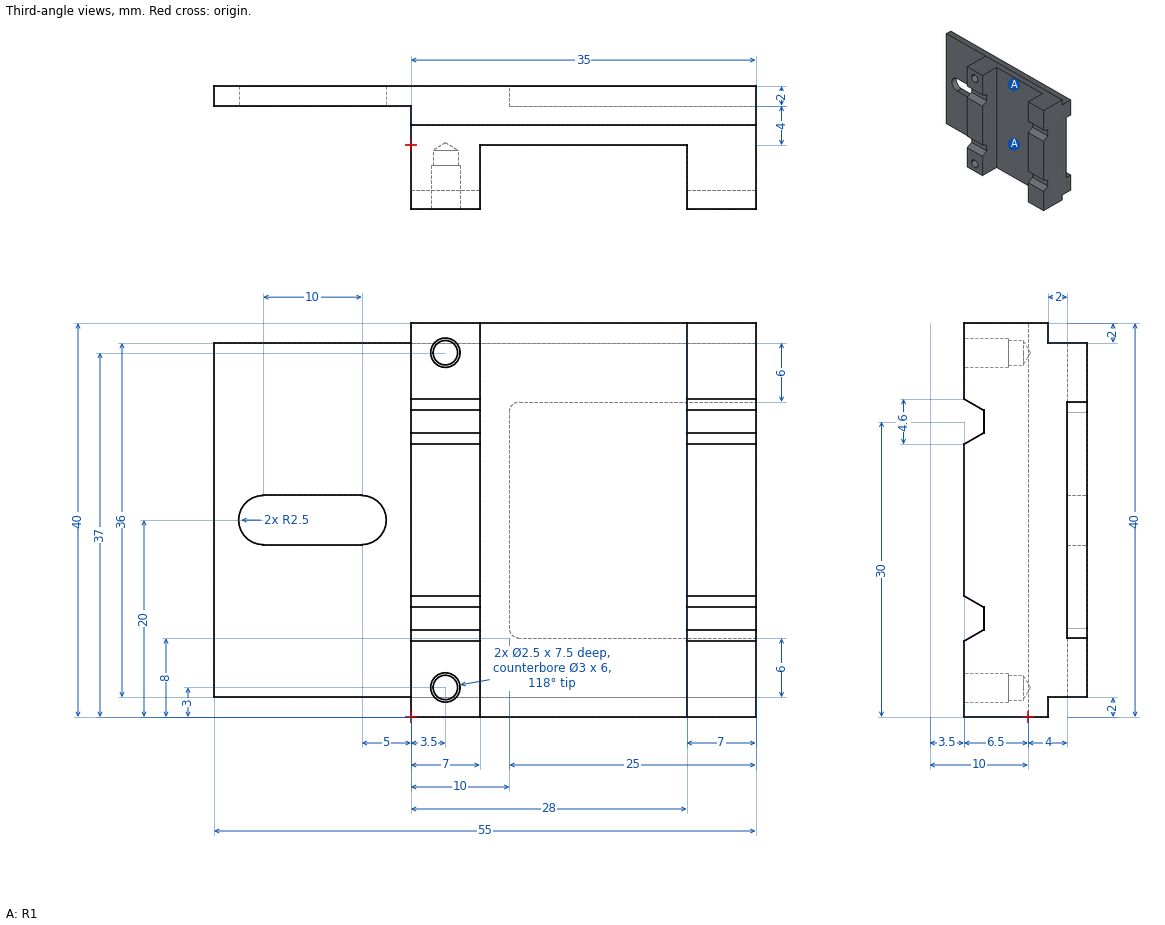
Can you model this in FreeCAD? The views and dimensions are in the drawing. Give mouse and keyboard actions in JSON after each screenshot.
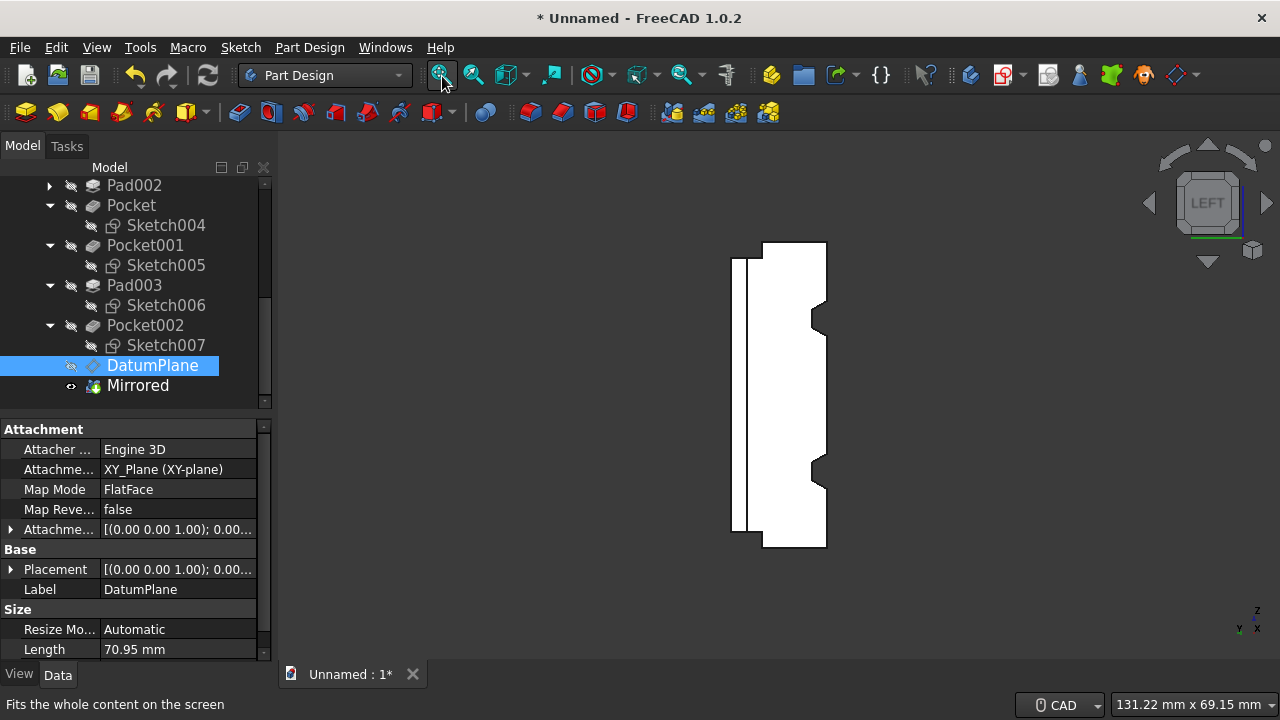
{"action": "key", "text": "0"}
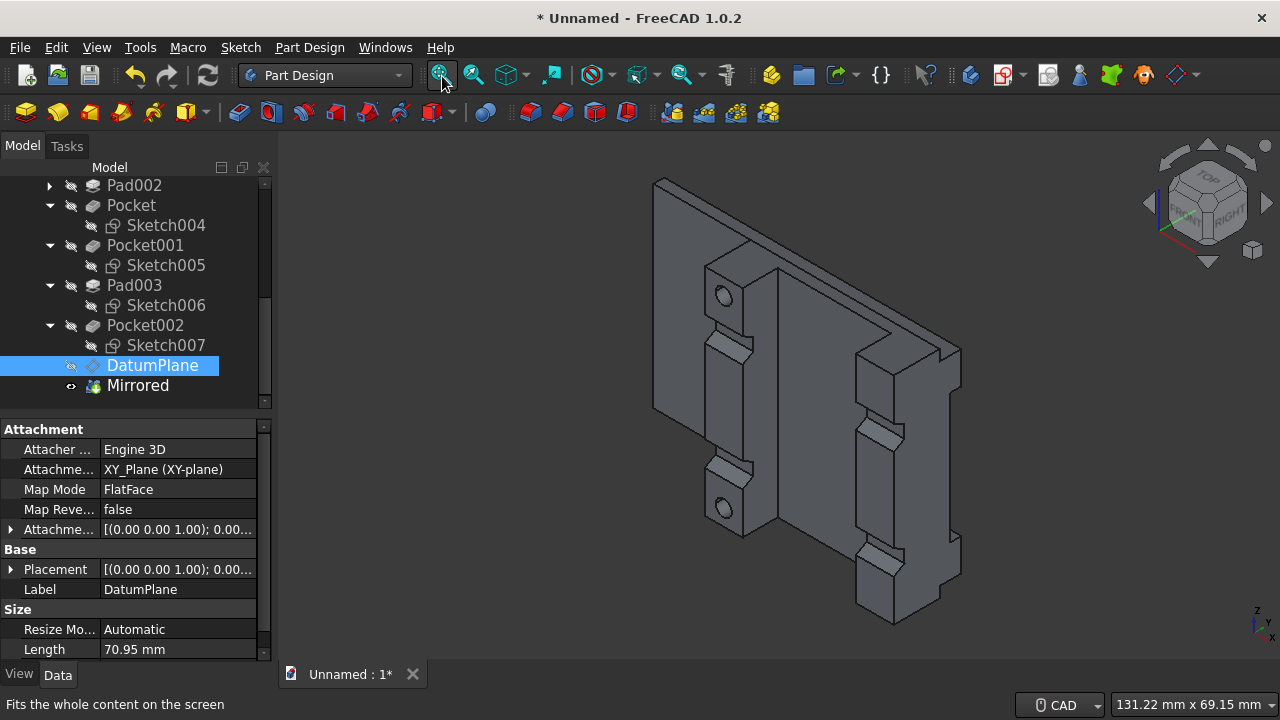
{"action": "scroll", "coordinate": [821, 311], "scroll_direction": "up", "scroll_amount": 5}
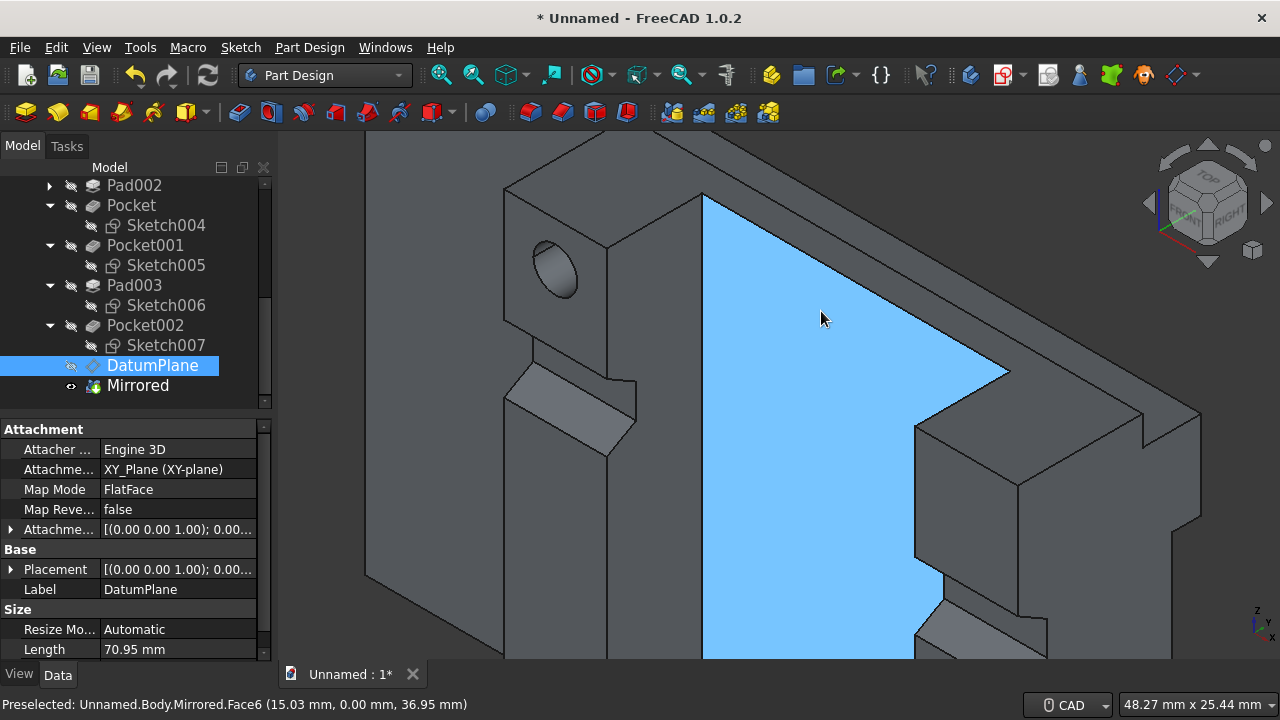
{"action": "left_click", "coordinate": [442, 76]}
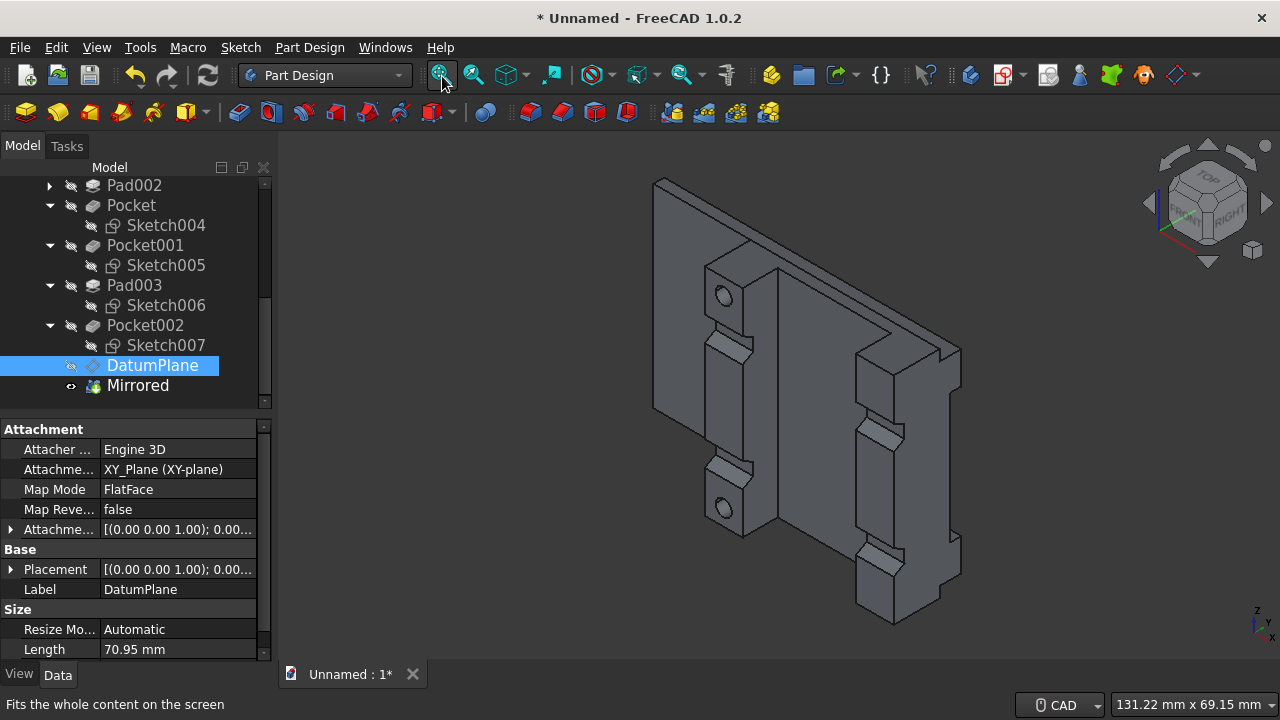
{"action": "key", "text": "2"}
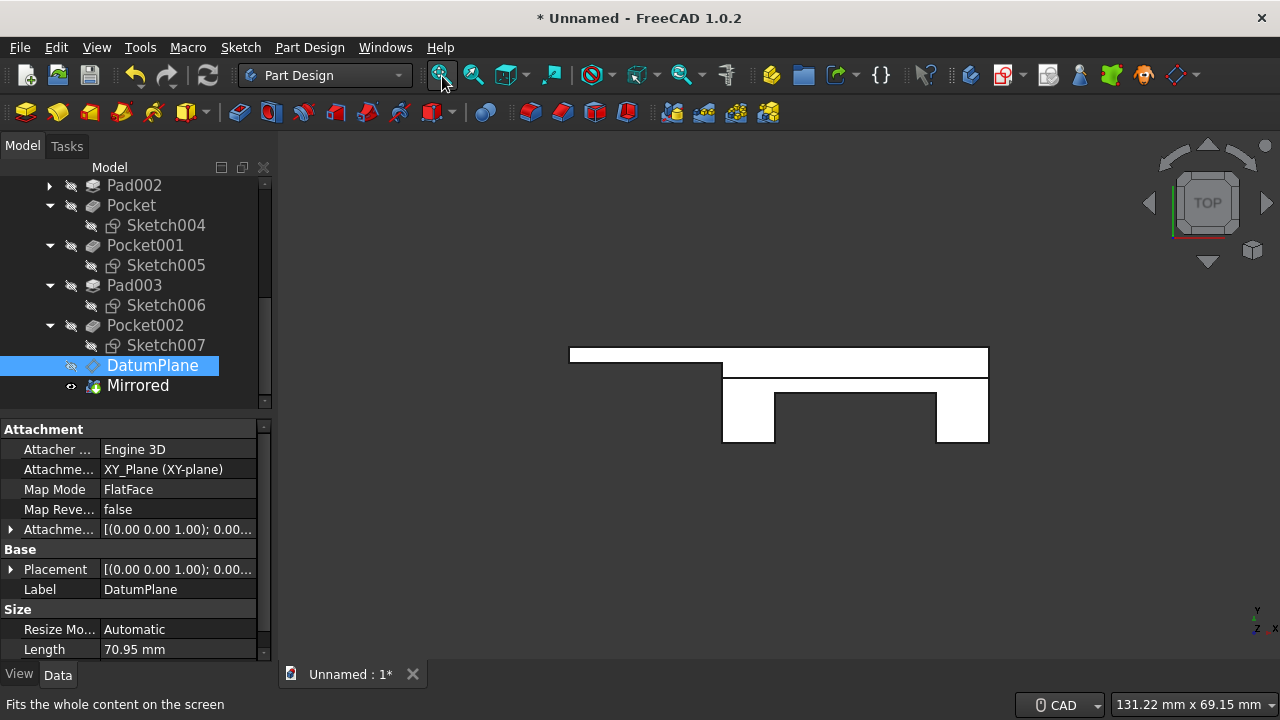
{"action": "left_click", "coordinate": [442, 76]}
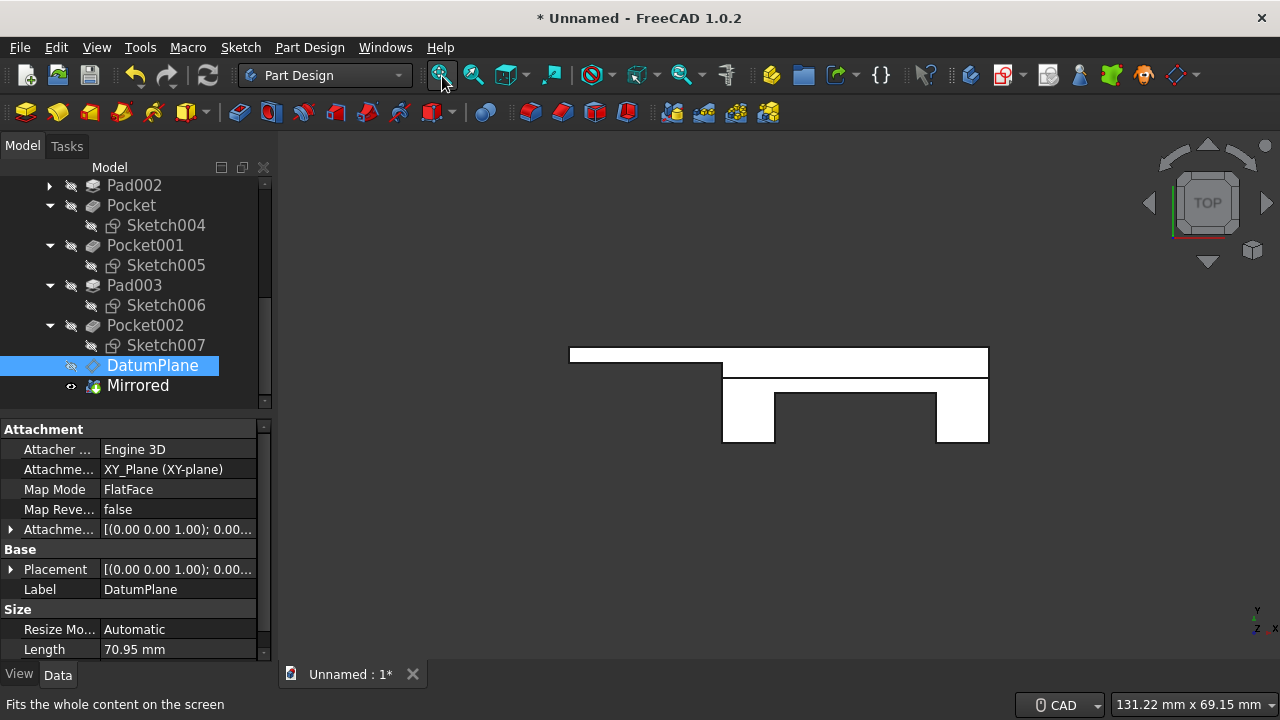
{"action": "scroll", "coordinate": [798, 354], "scroll_direction": "up", "scroll_amount": 5}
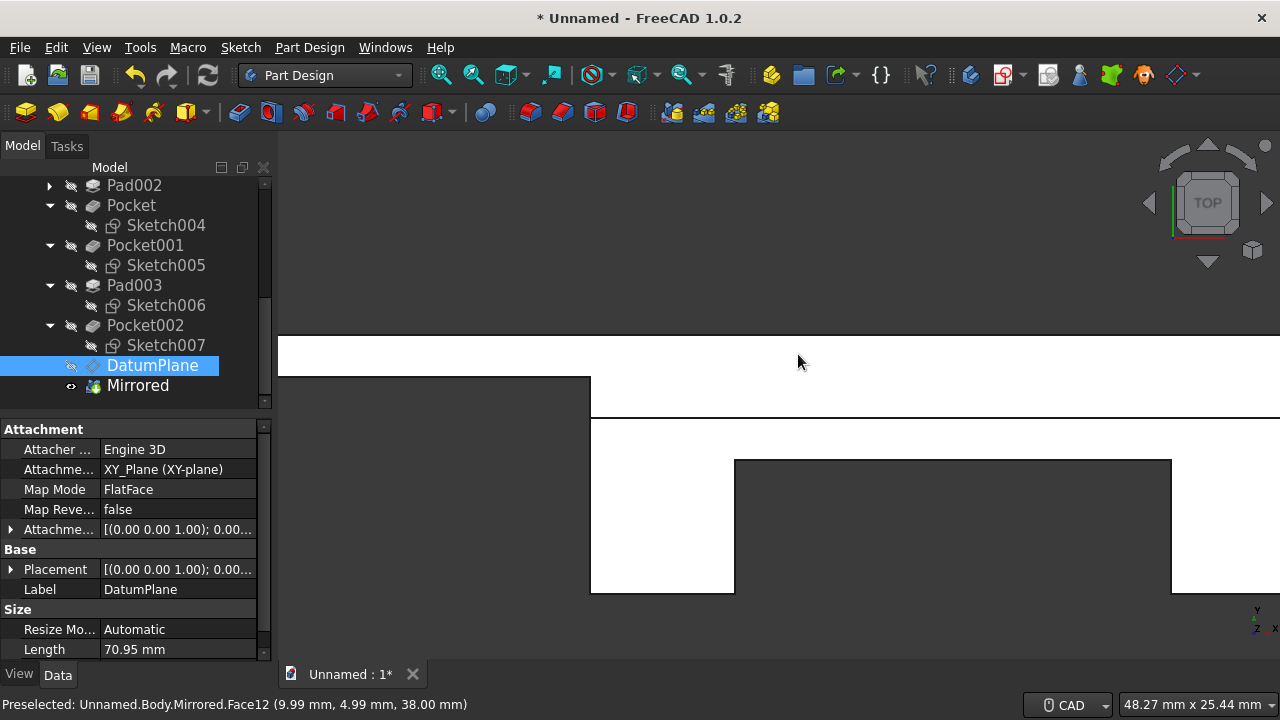
{"action": "left_click", "coordinate": [442, 76]}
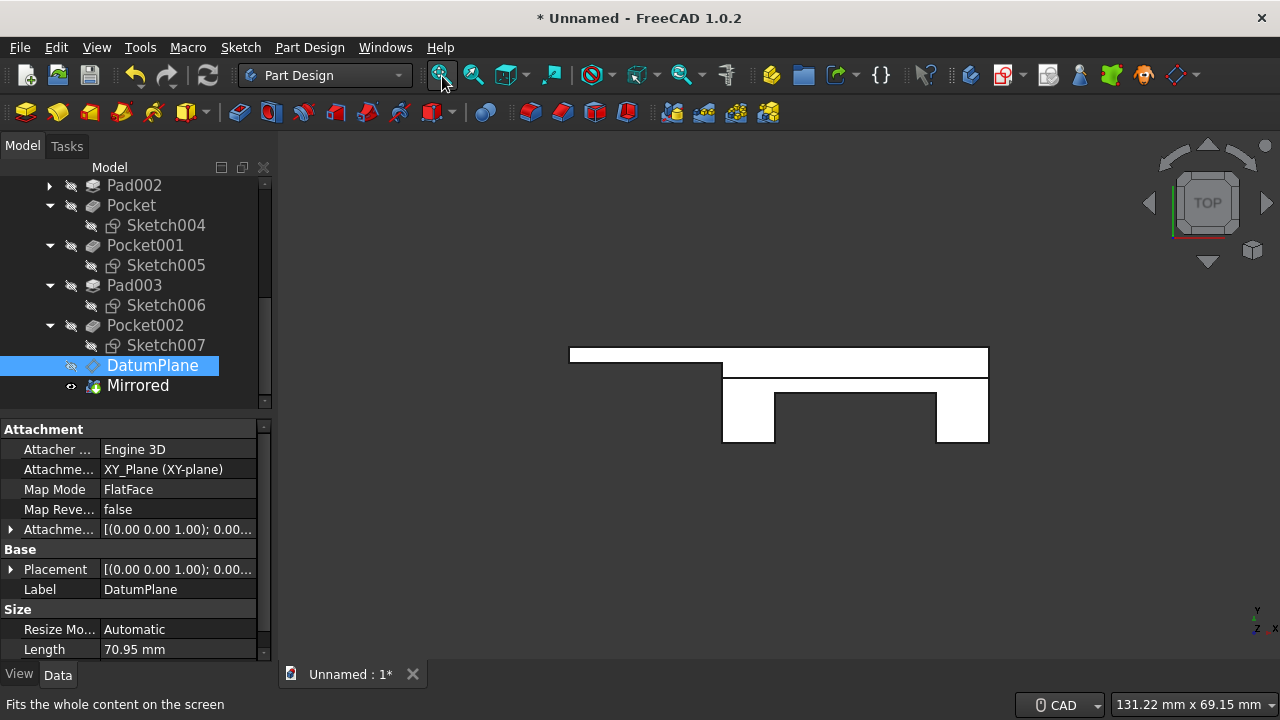
{"action": "key", "text": "1"}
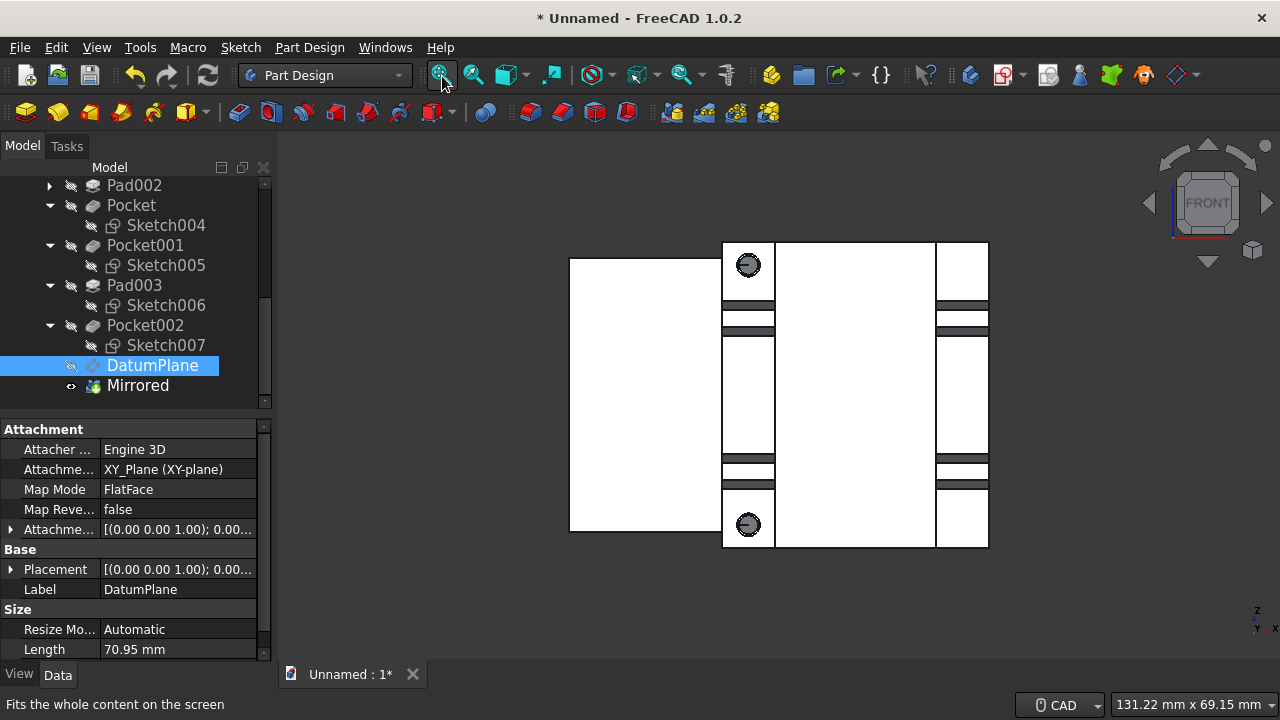
{"action": "scroll", "coordinate": [798, 302], "scroll_direction": "up", "scroll_amount": 5}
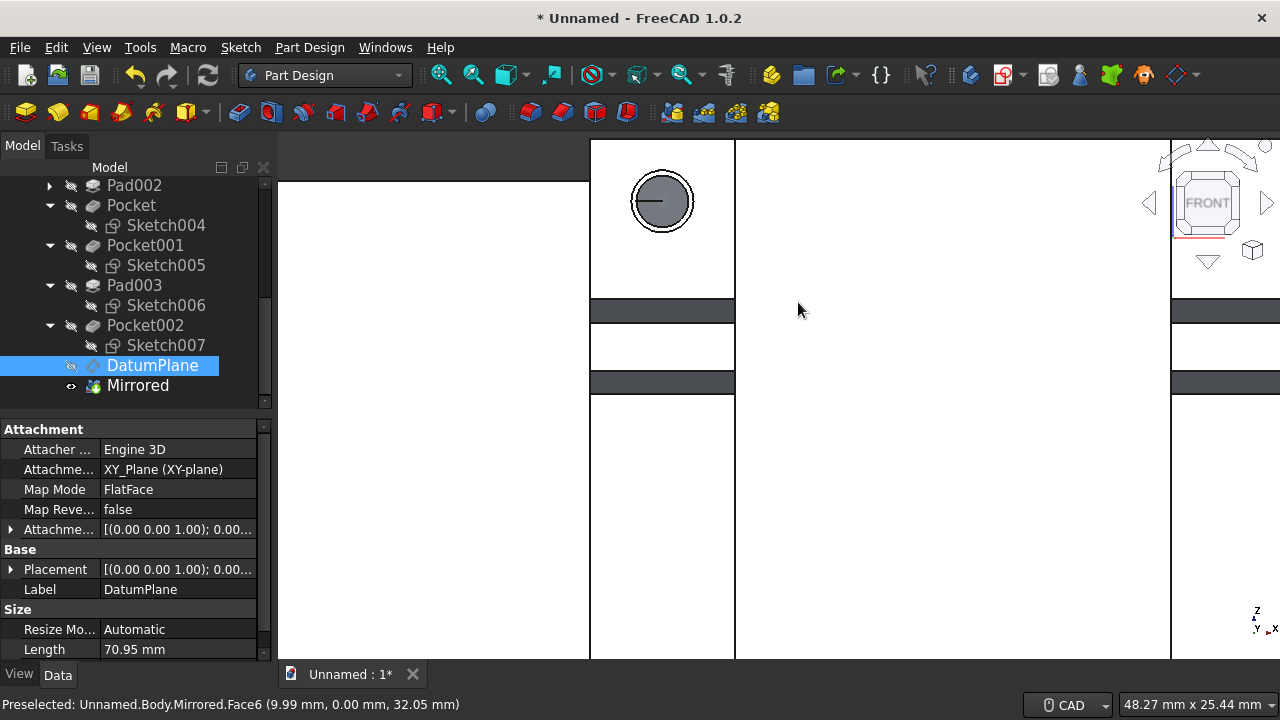
{"action": "left_click", "coordinate": [442, 76]}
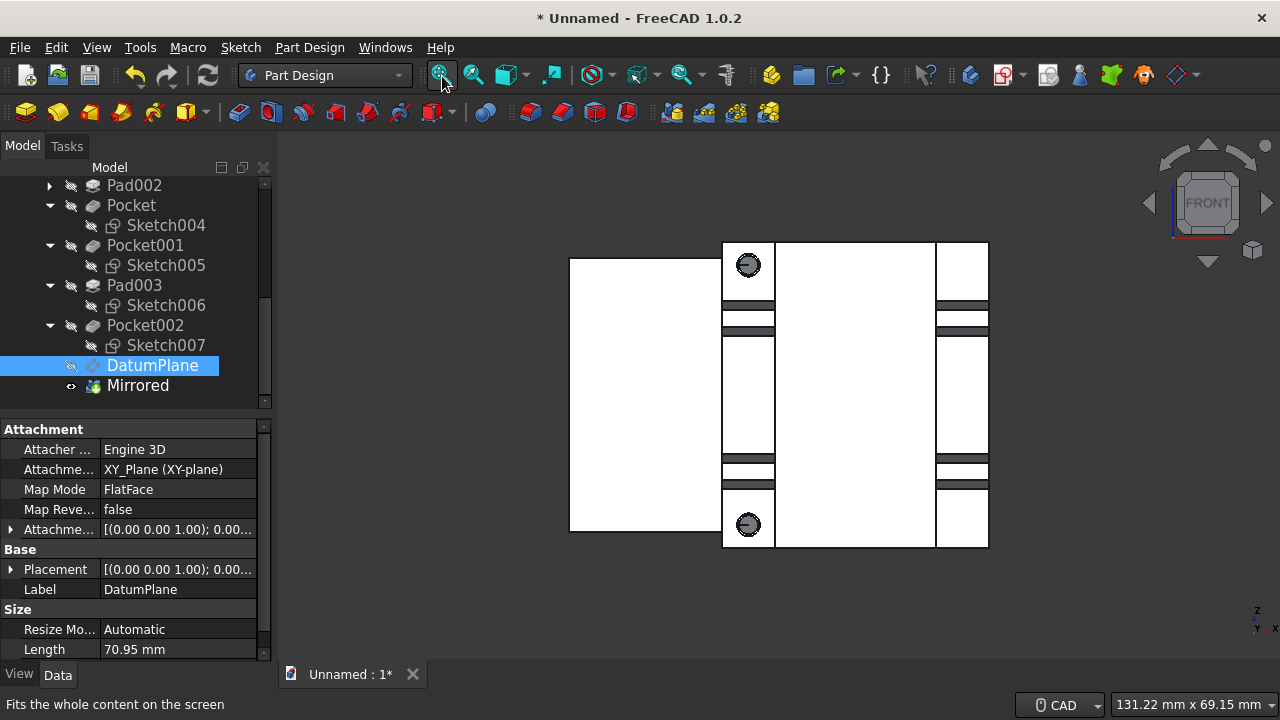
{"action": "key", "text": "3"}